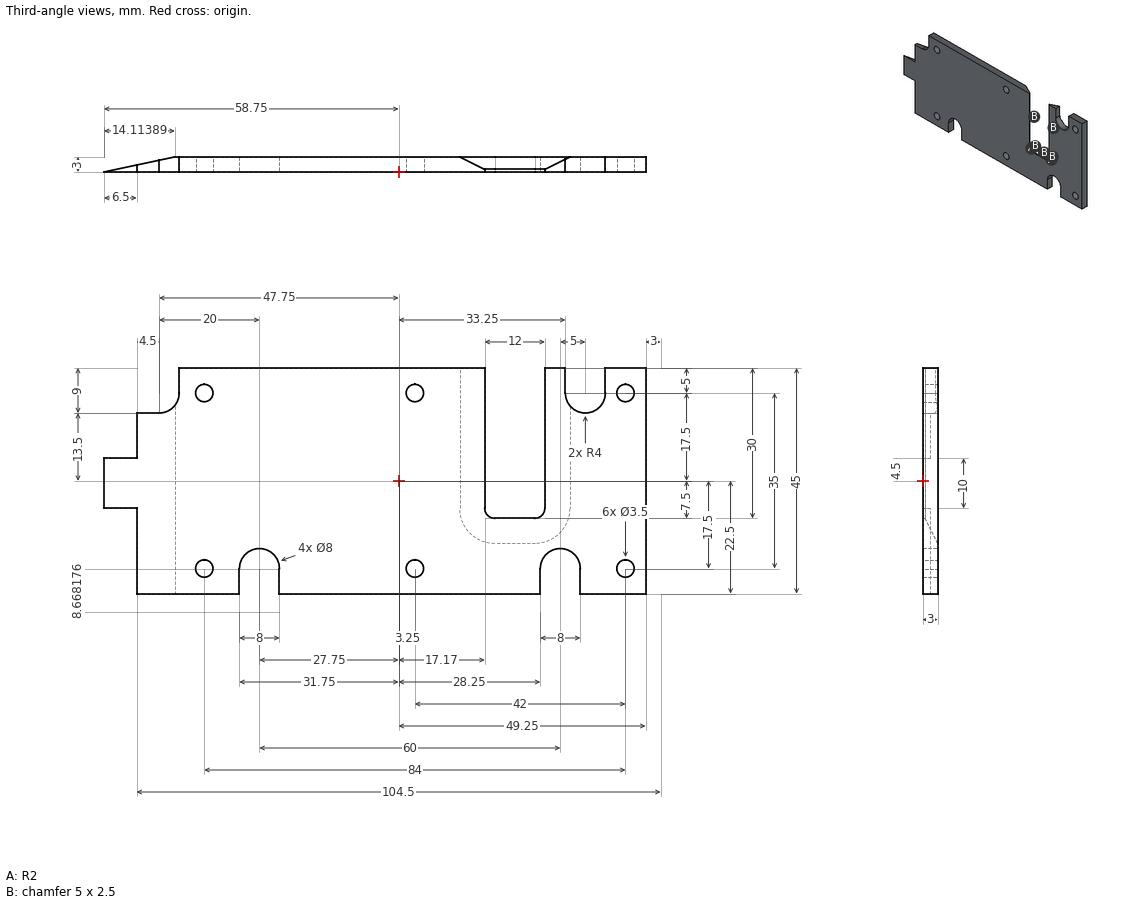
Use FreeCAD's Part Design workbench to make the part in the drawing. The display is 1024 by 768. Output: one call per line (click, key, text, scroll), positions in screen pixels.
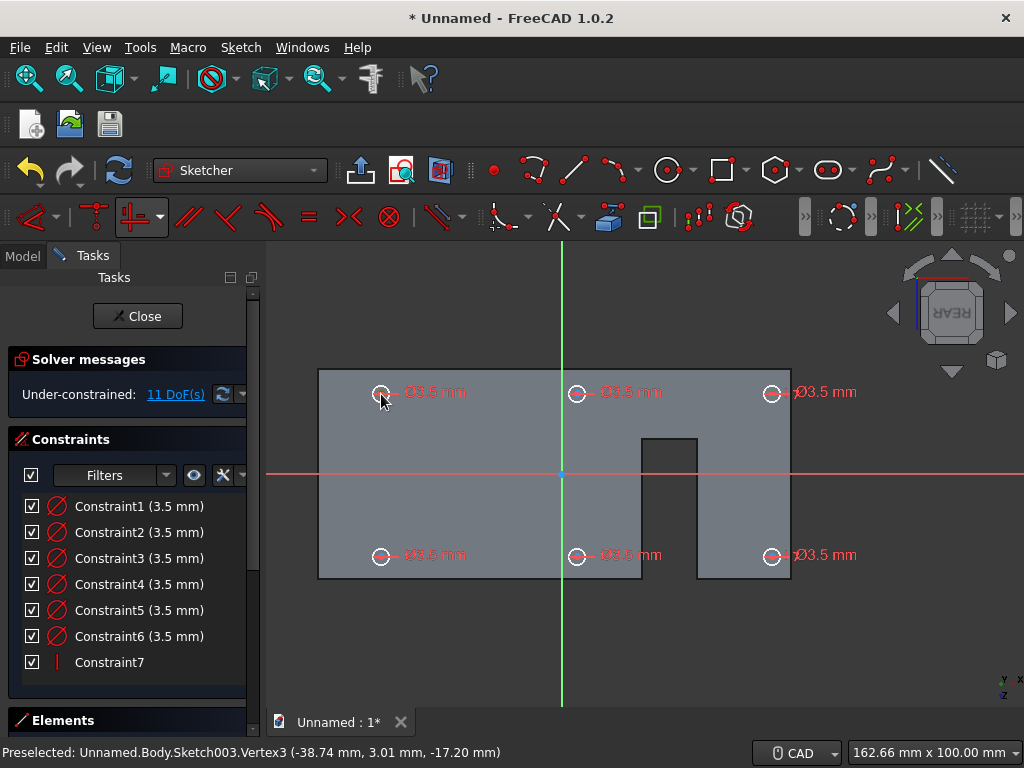
click(162, 218)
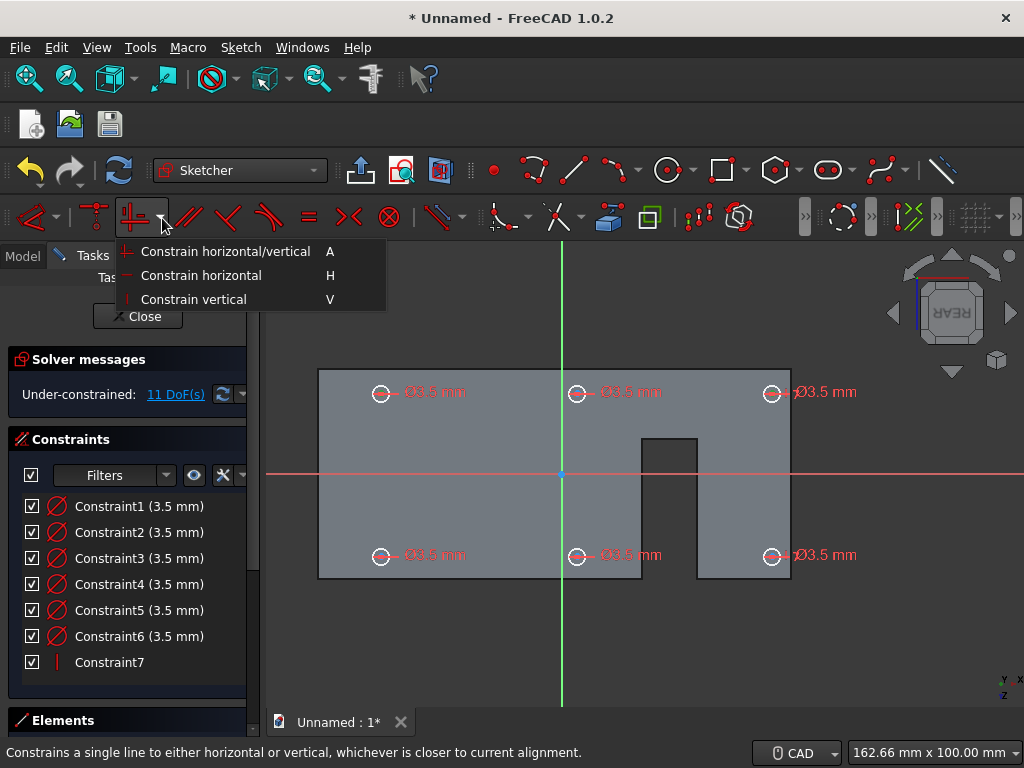
click(251, 275)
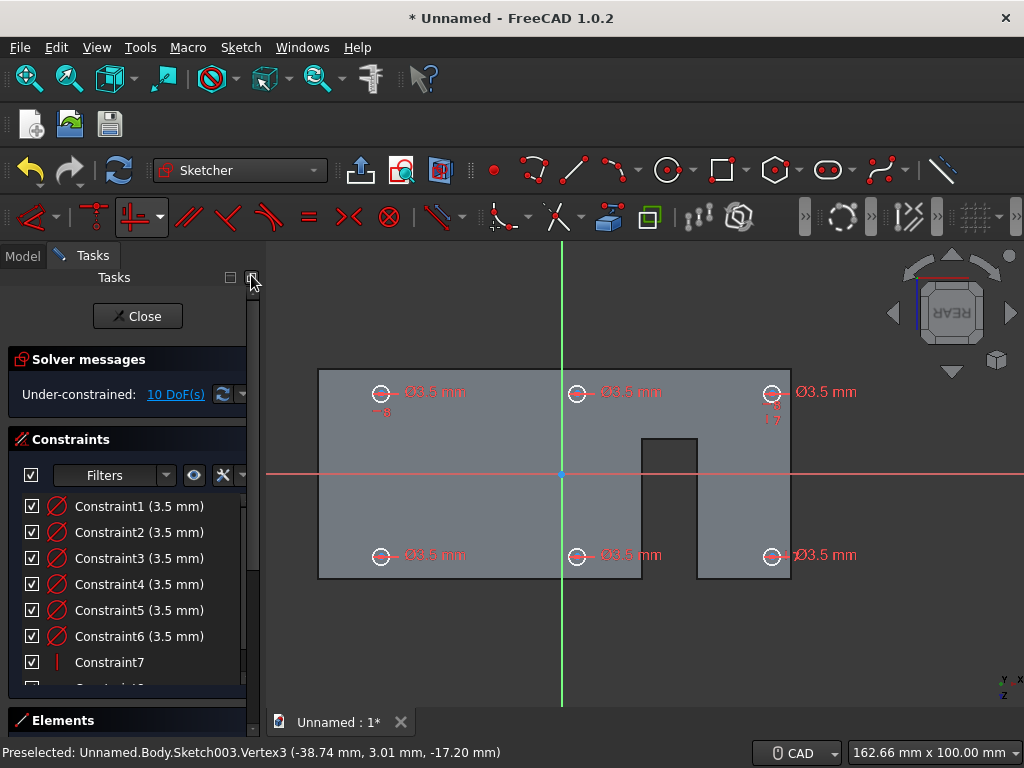
click(772, 394)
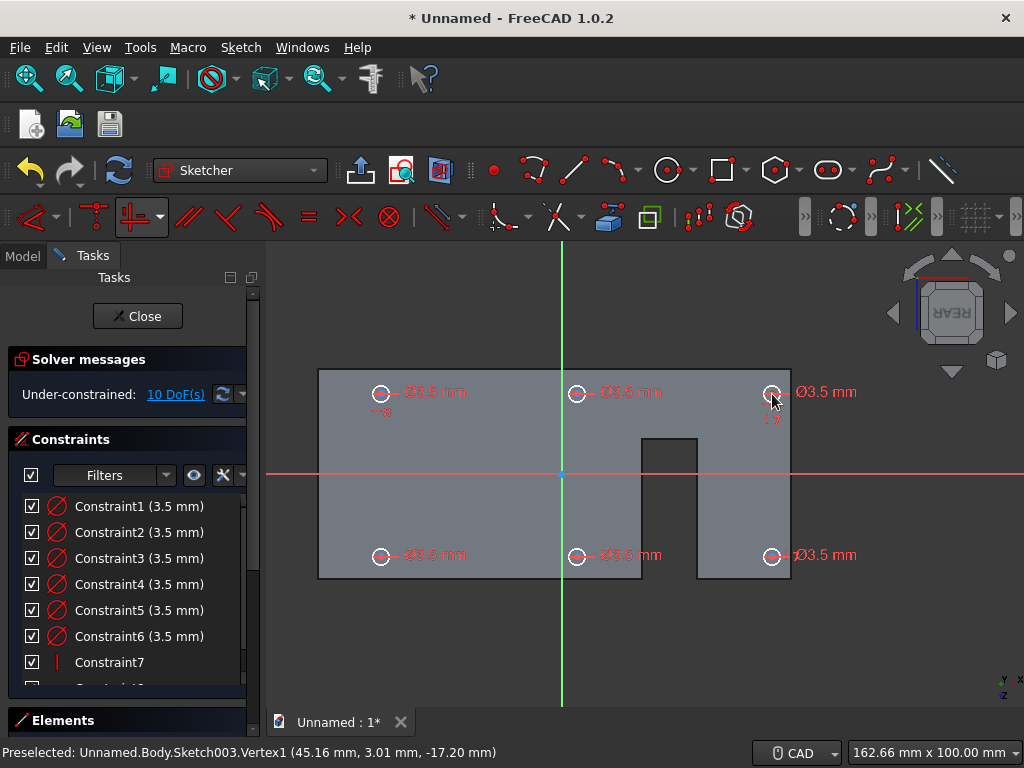
click(577, 394)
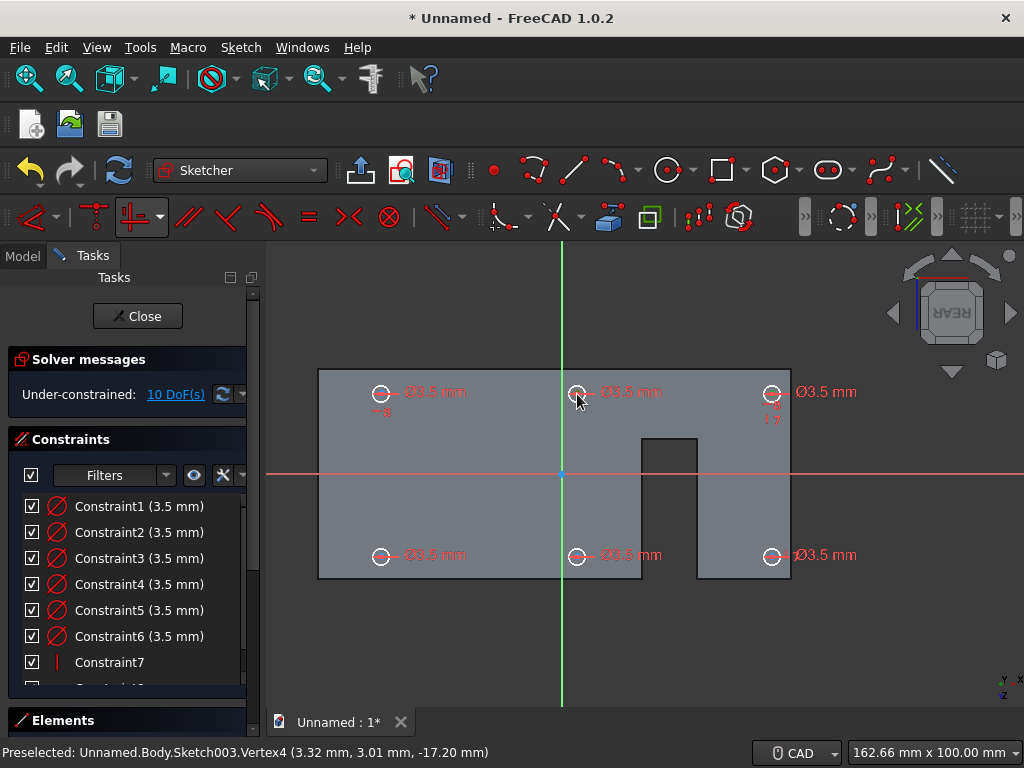
key(h)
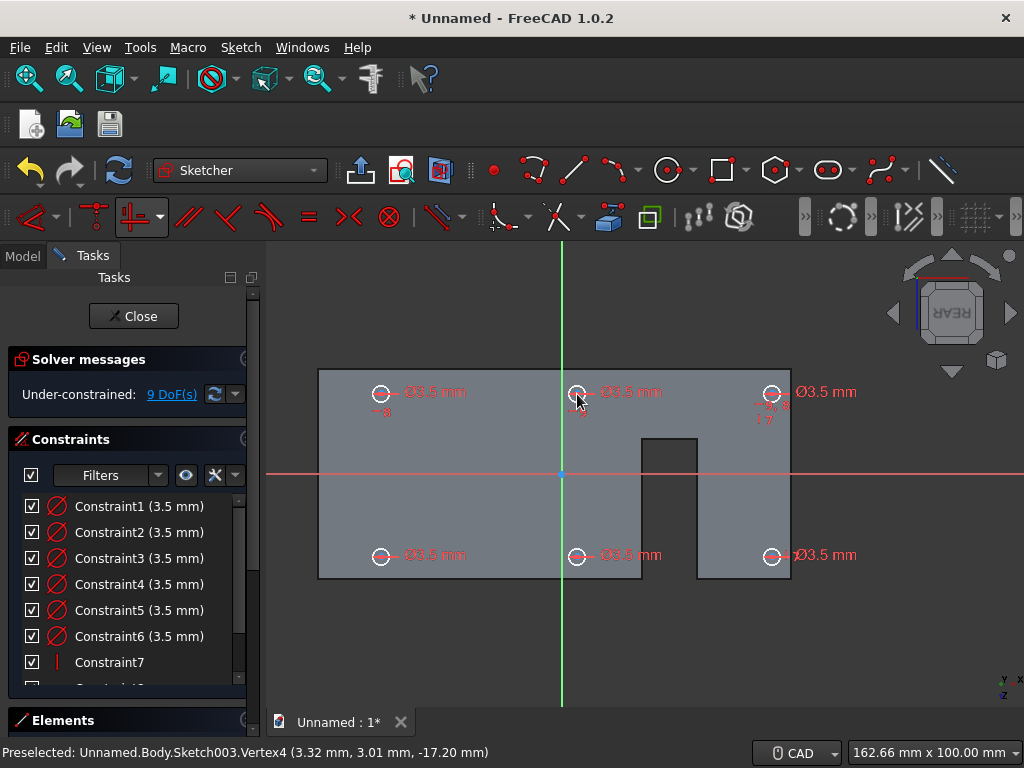
click(381, 394)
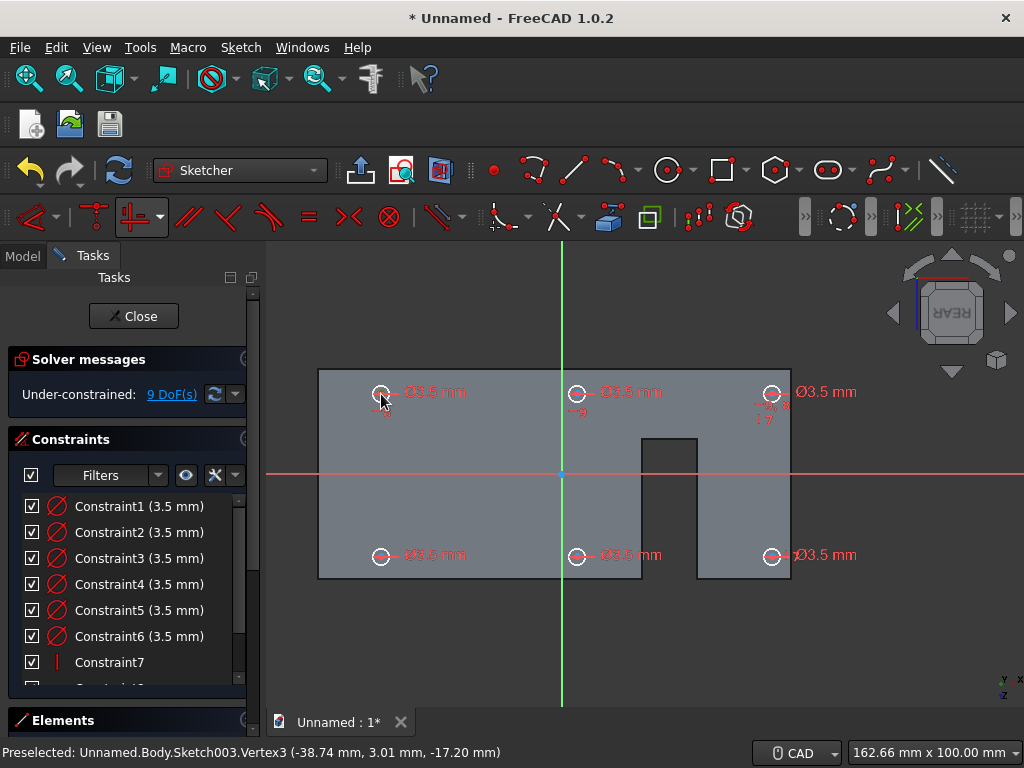
click(381, 557)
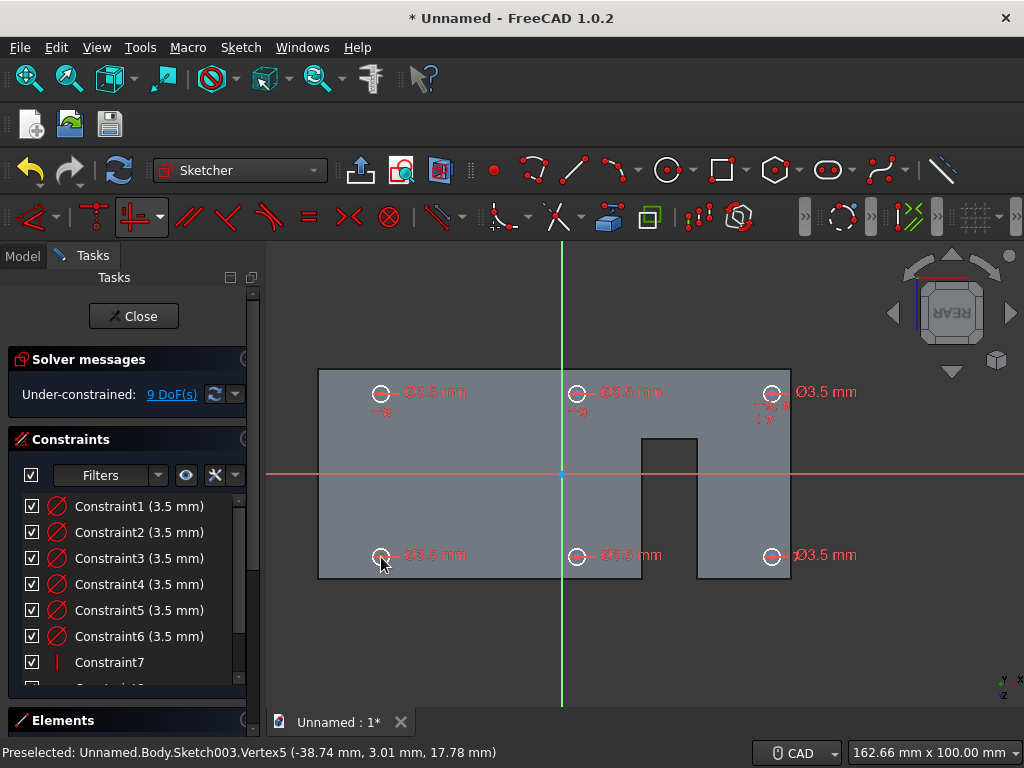
key(v)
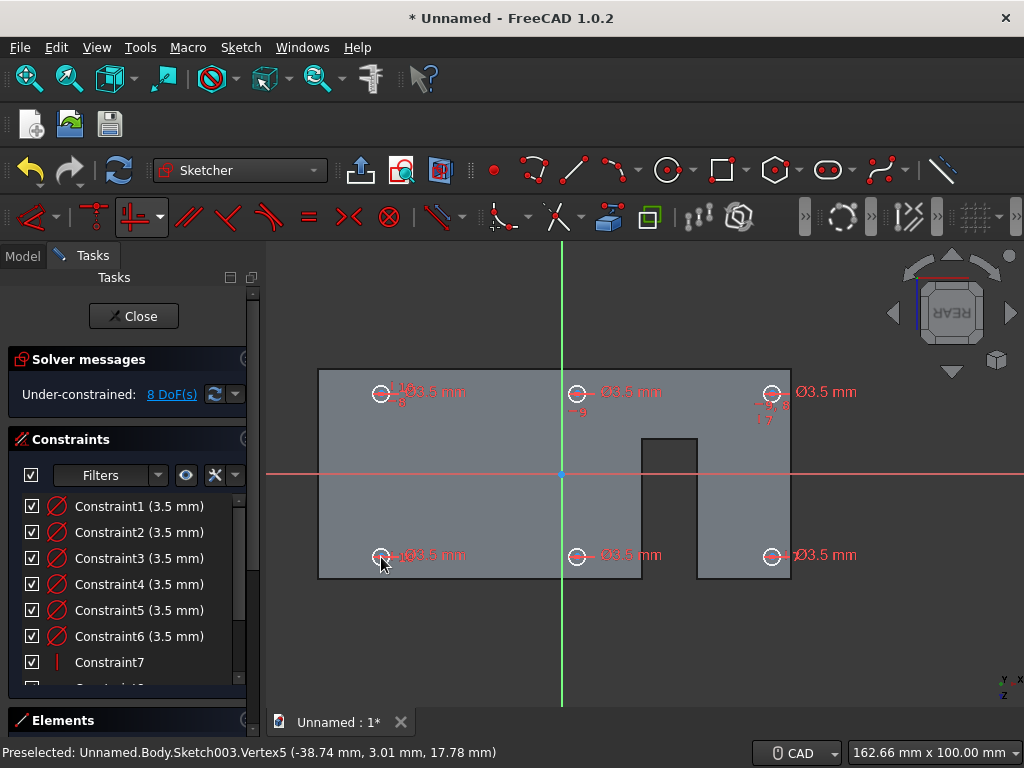
click(772, 557)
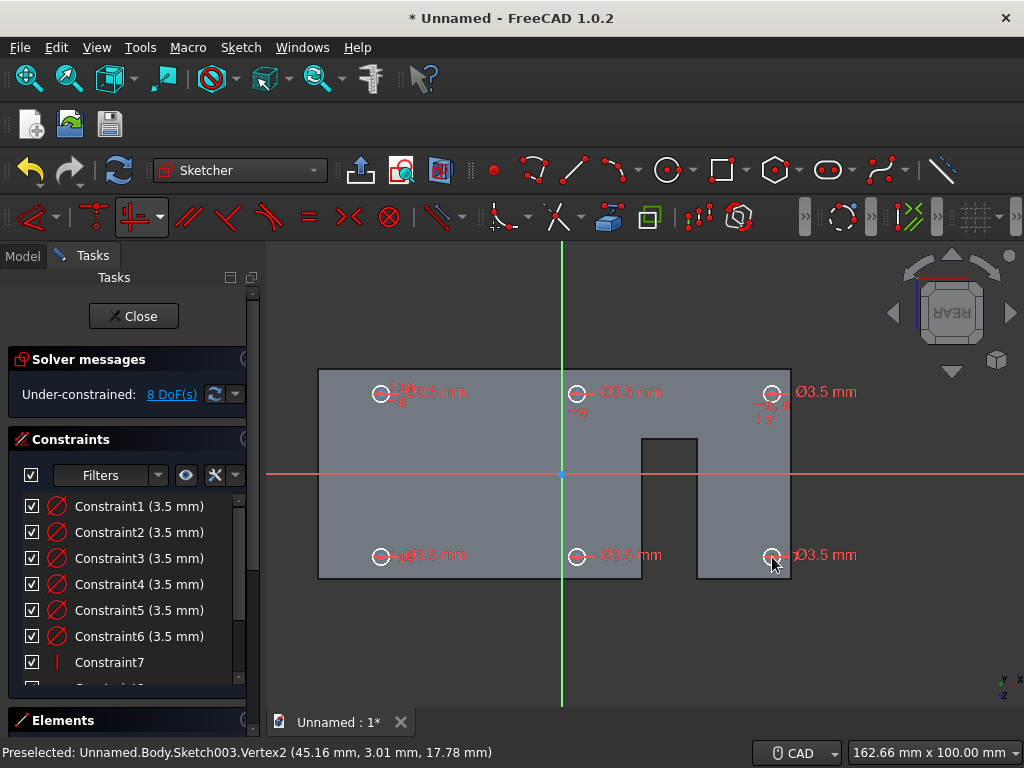
click(381, 557)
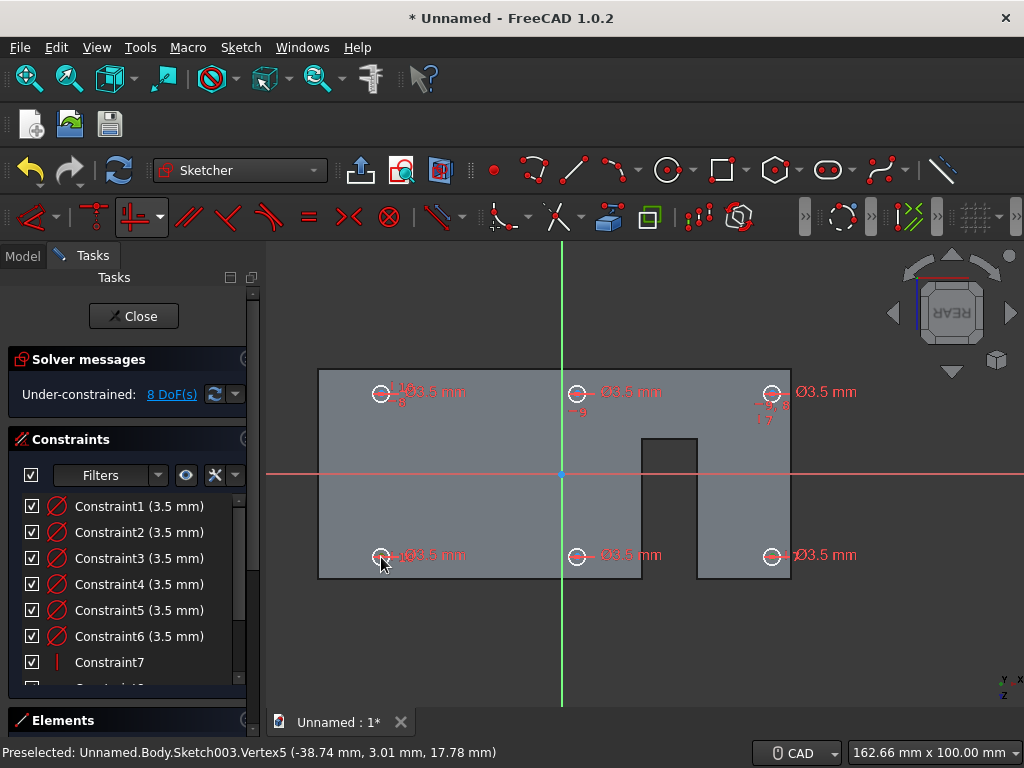
key(h)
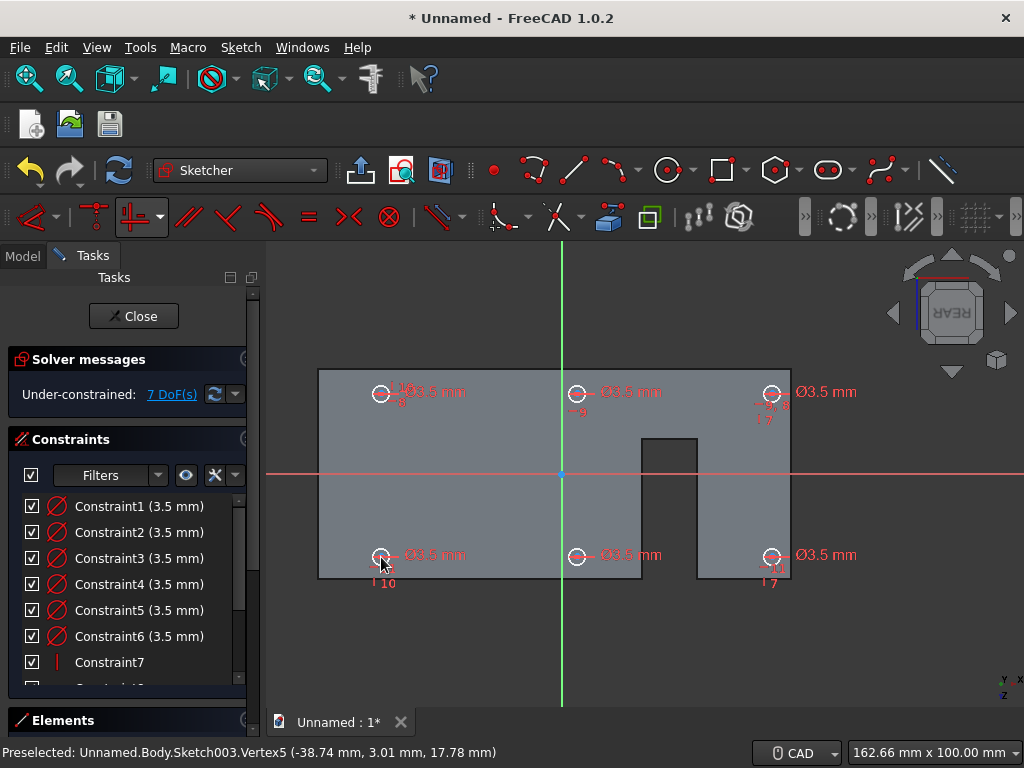
click(577, 394)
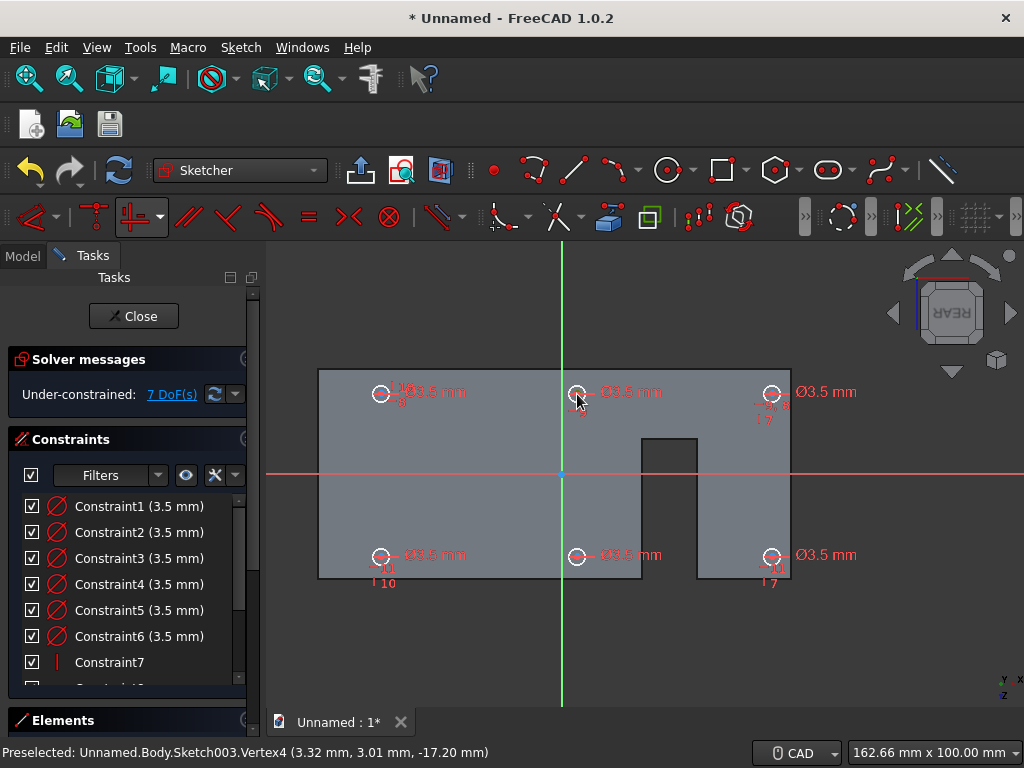
click(577, 557)